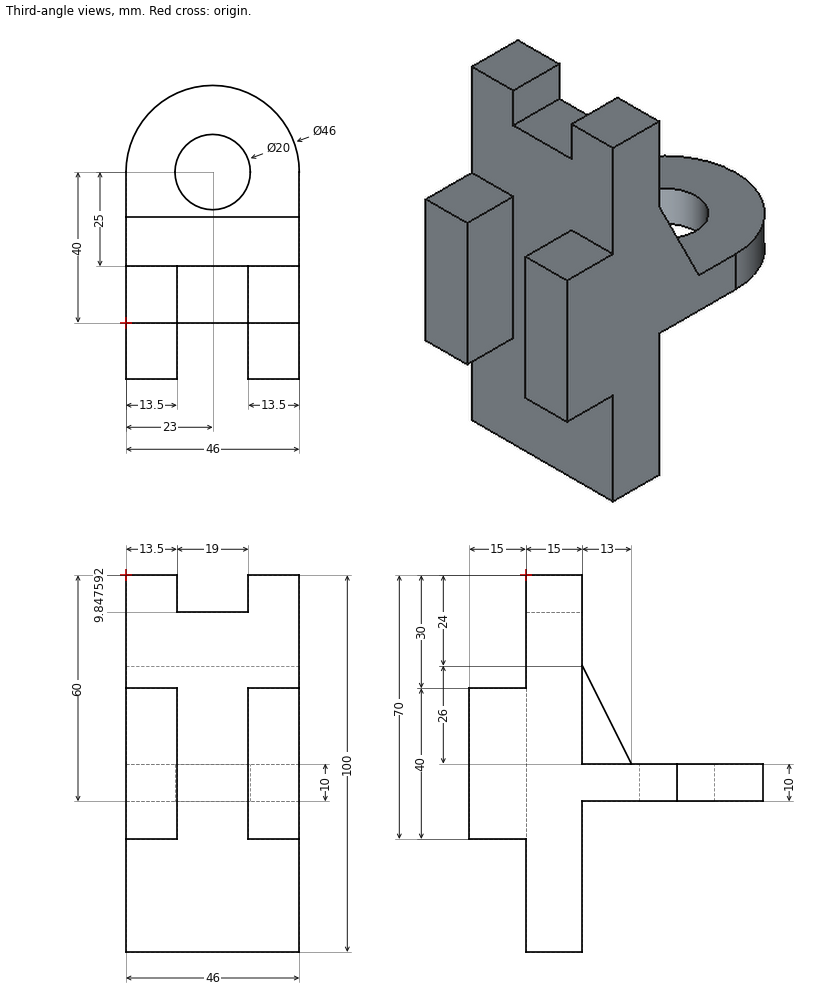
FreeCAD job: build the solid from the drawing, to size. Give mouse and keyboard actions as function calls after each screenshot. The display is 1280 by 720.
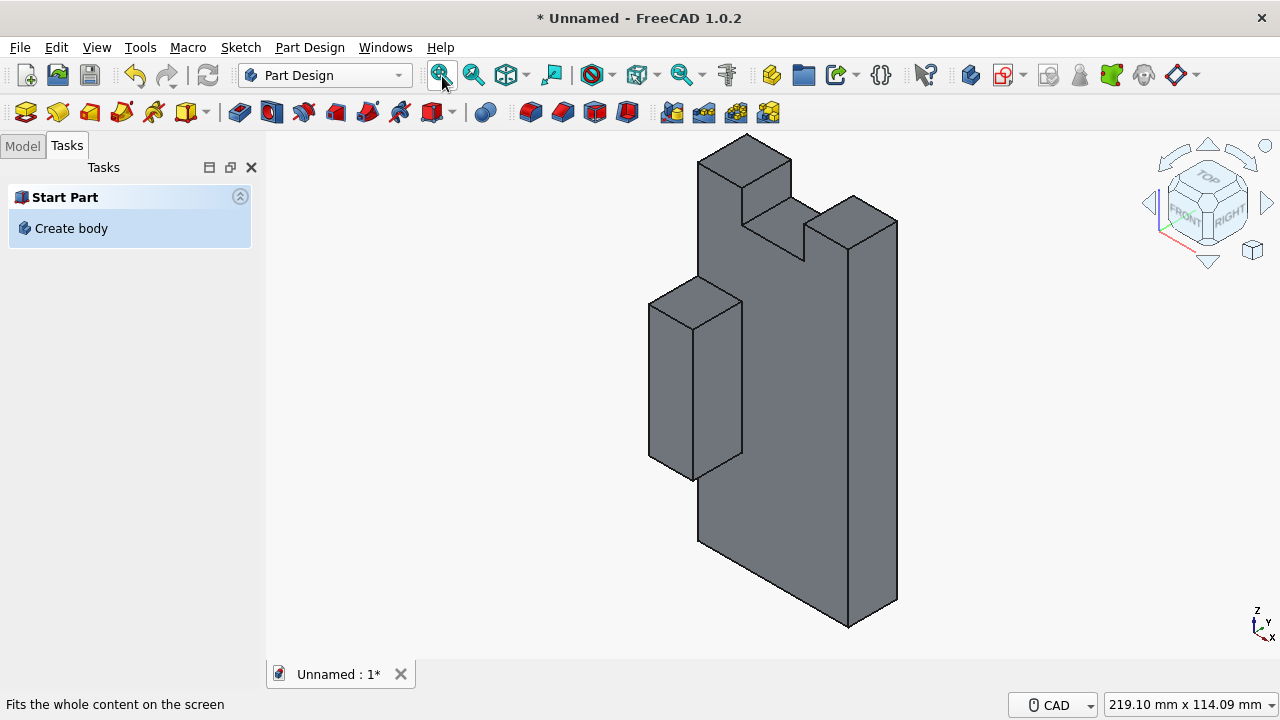
click(873, 369)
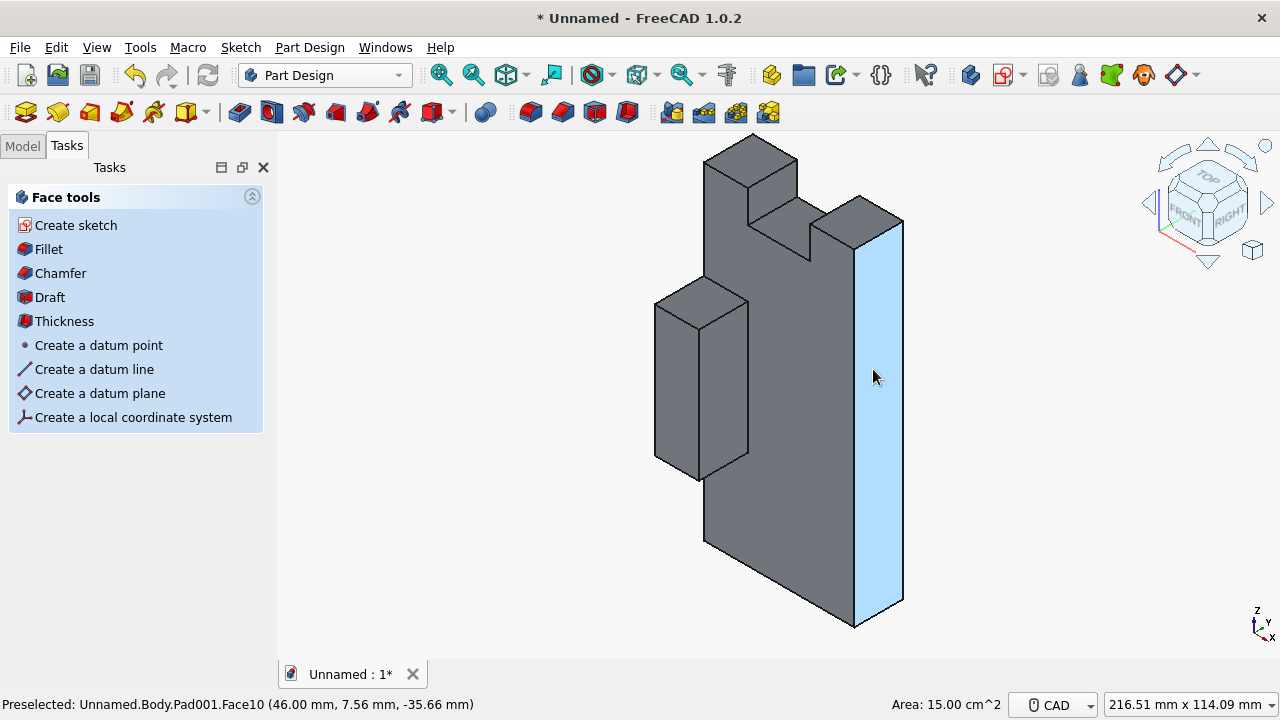
click(1004, 76)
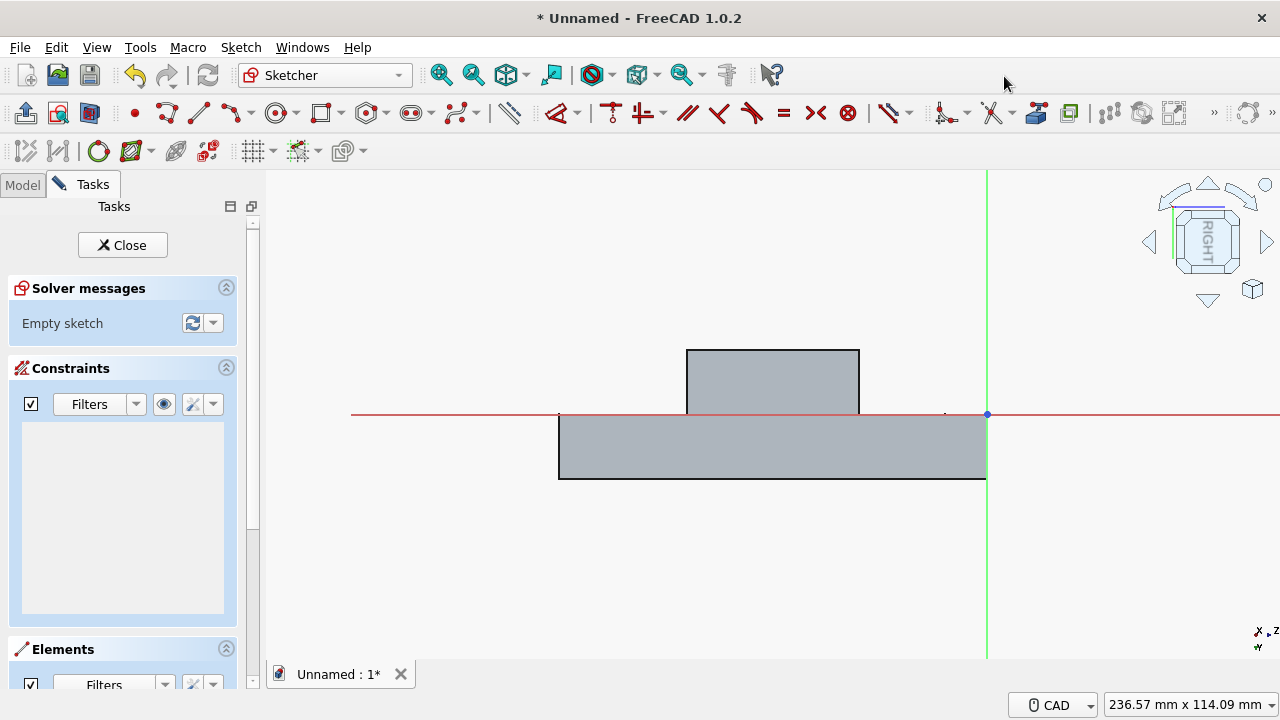
scroll(999, 343, up, 3)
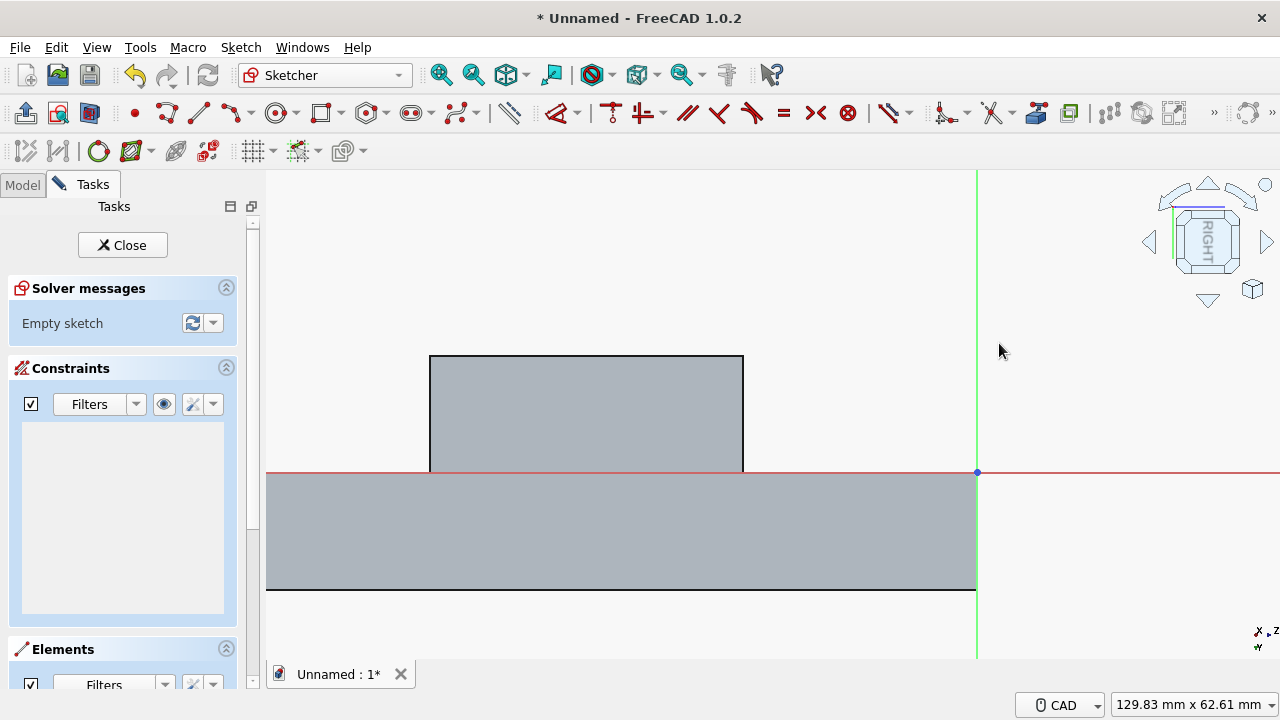
key(g)
key(r)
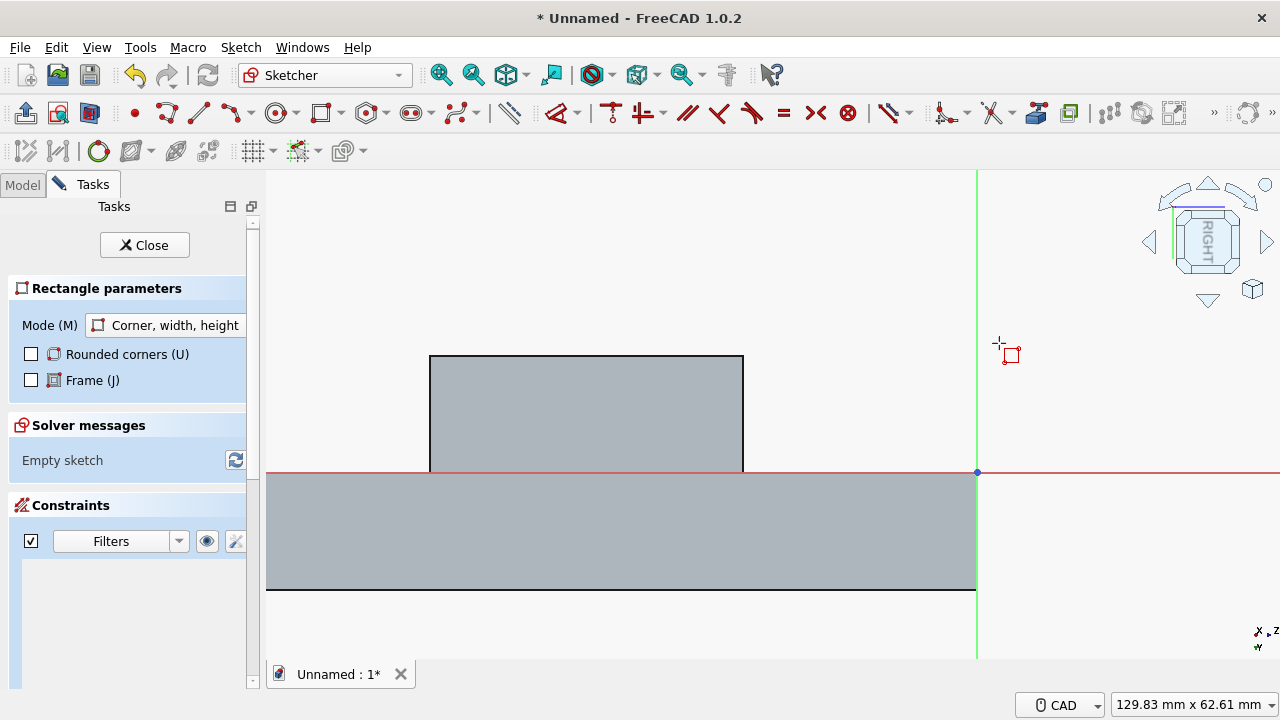
click(430, 356)
click(743, 473)
key(Escape)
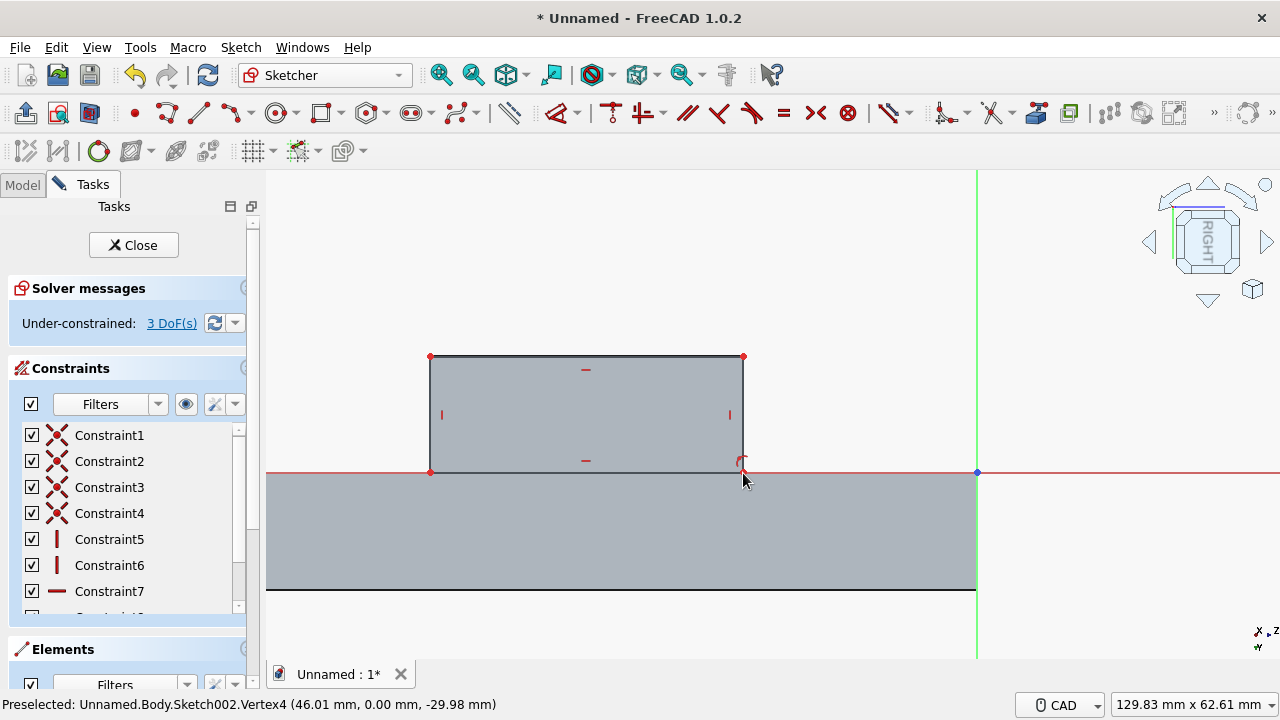
key(d)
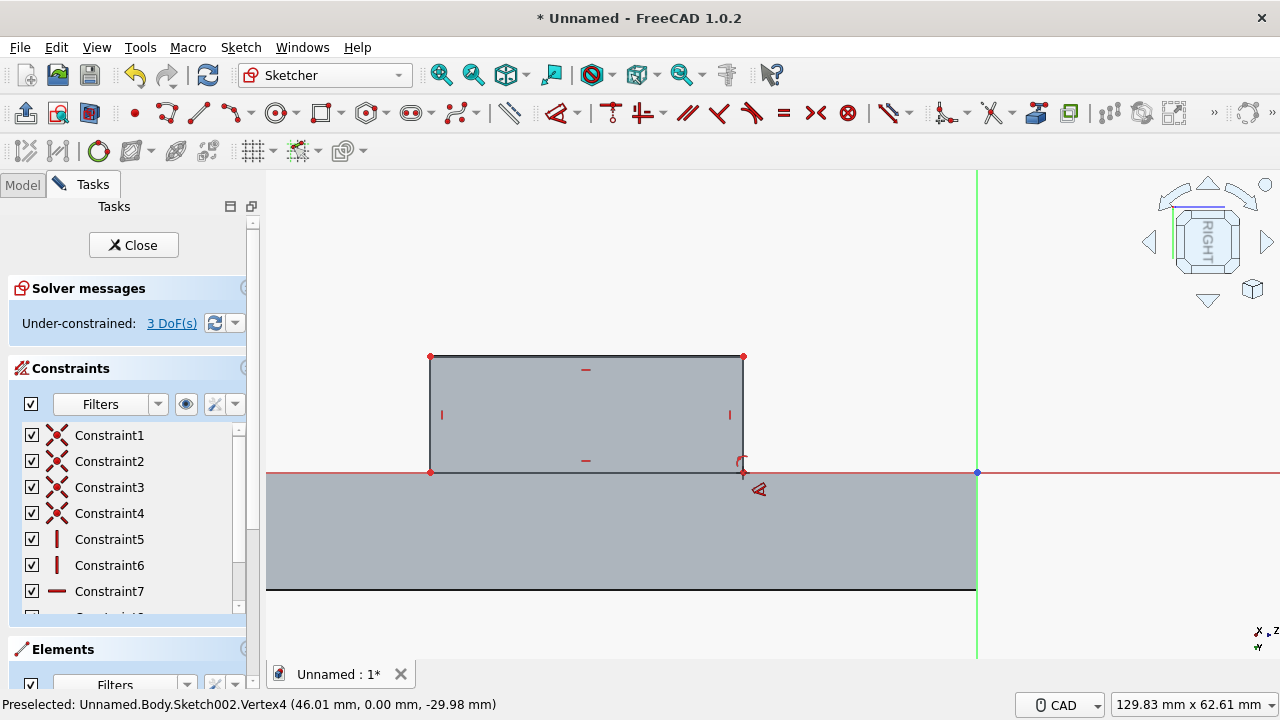
click(430, 392)
click(396, 415)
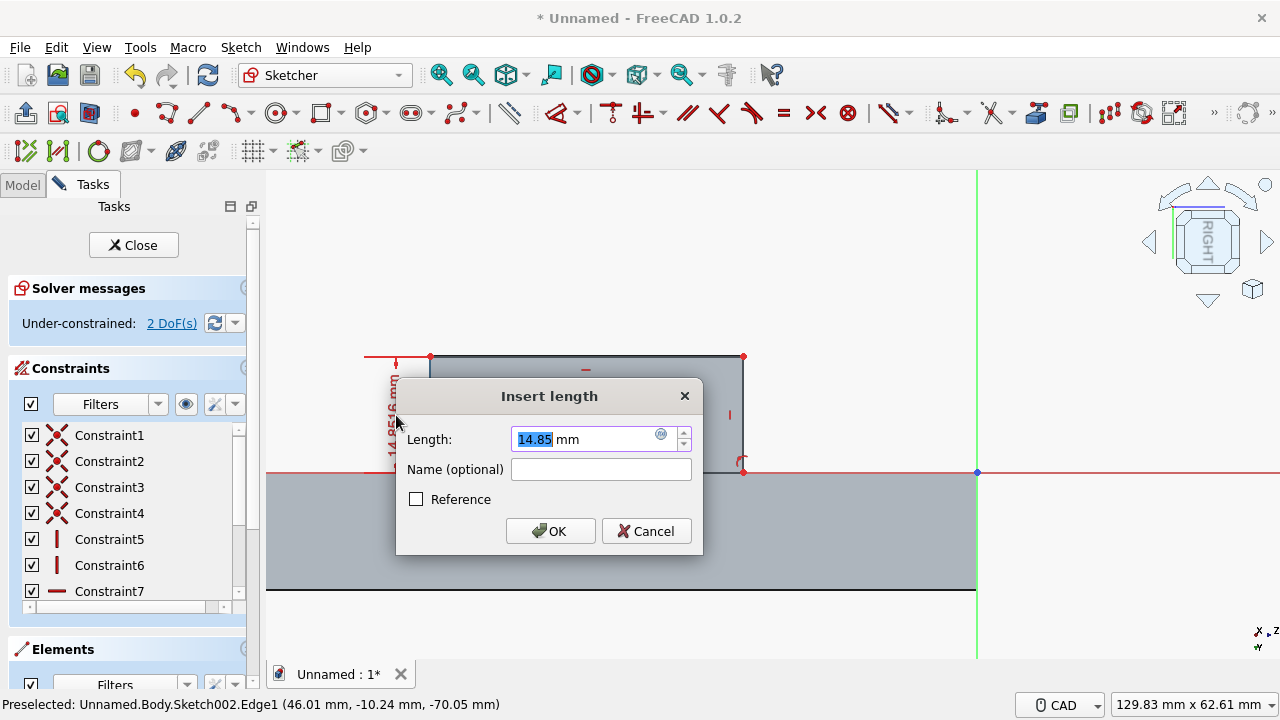
text(15)
key(Return)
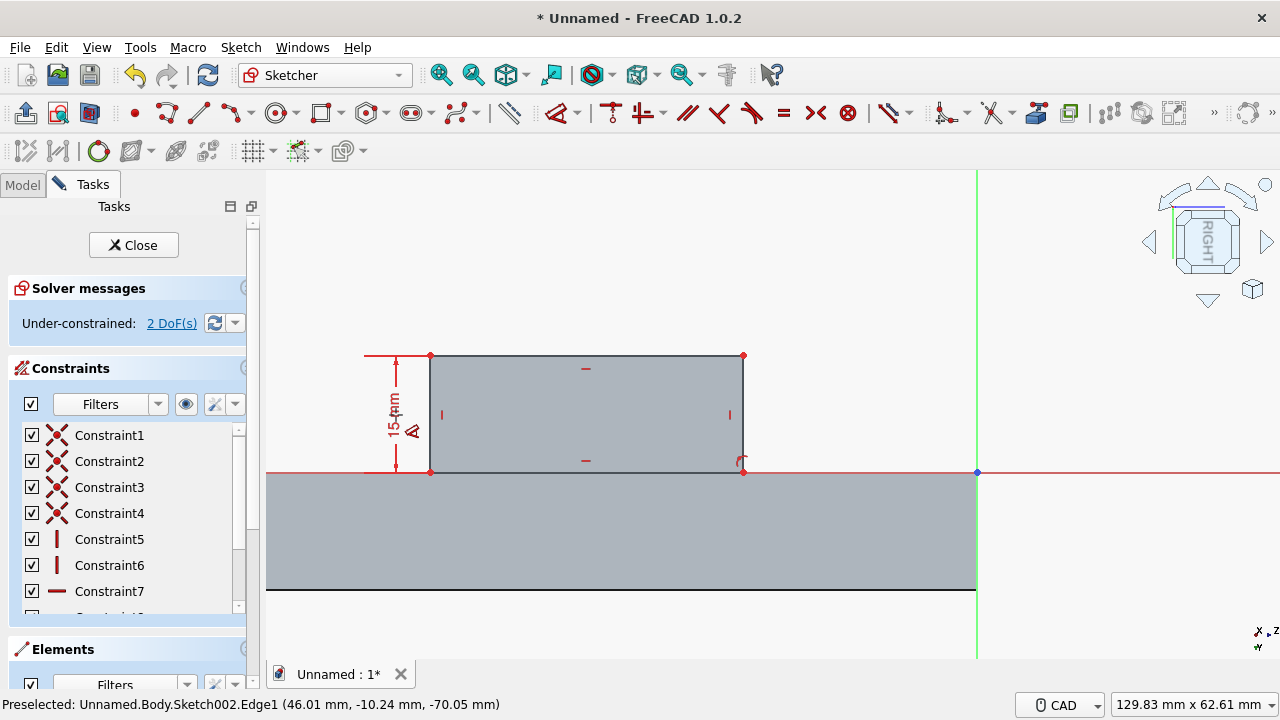
click(524, 473)
click(586, 507)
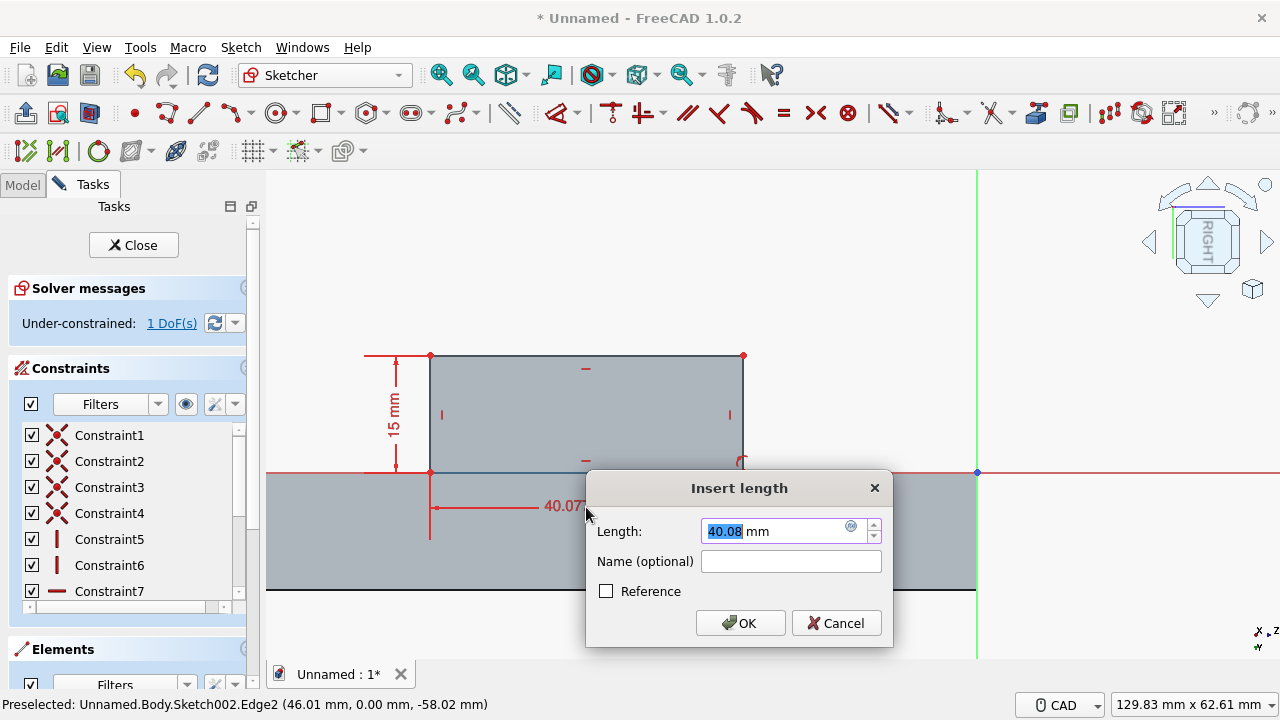
text(40)
key(Return)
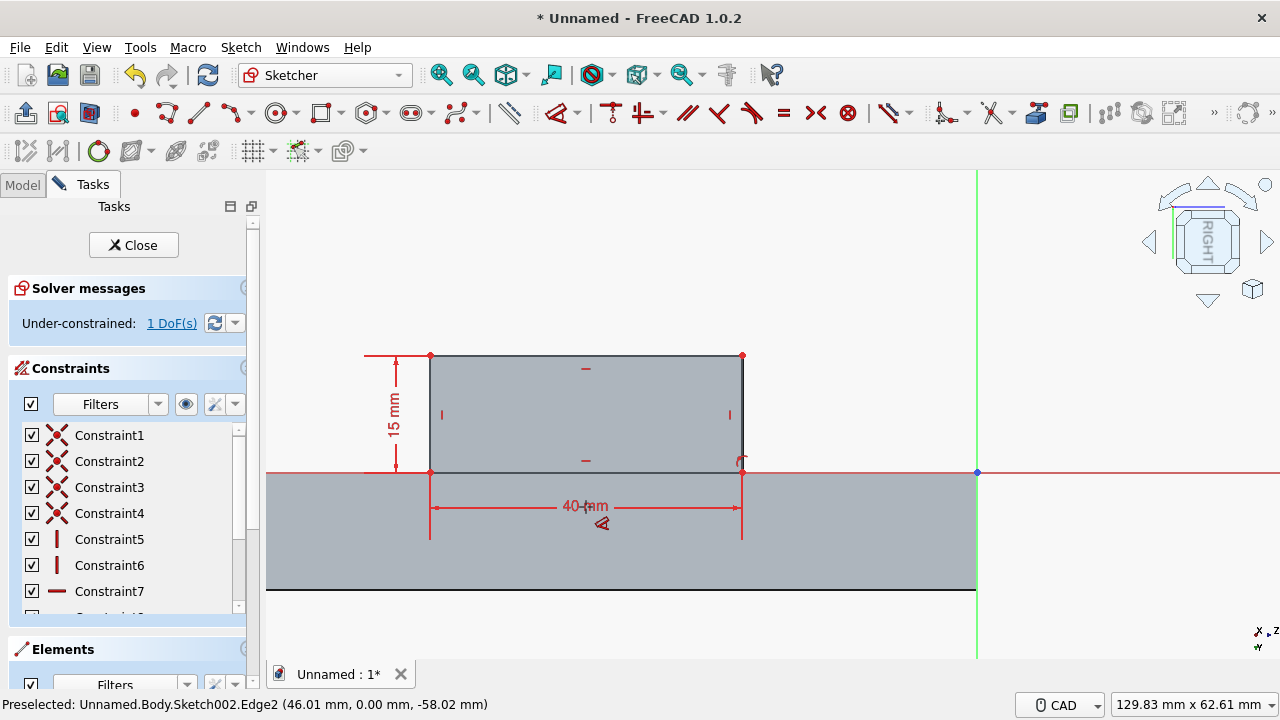
click(430, 356)
click(704, 507)